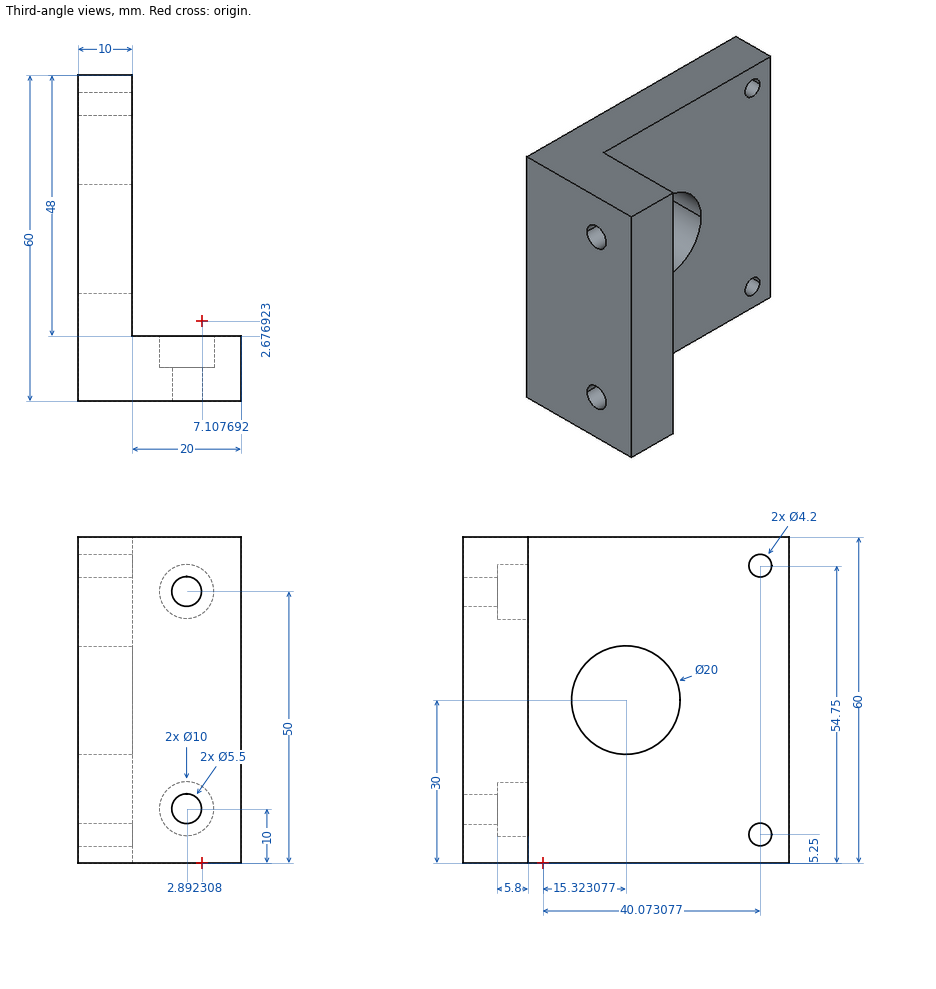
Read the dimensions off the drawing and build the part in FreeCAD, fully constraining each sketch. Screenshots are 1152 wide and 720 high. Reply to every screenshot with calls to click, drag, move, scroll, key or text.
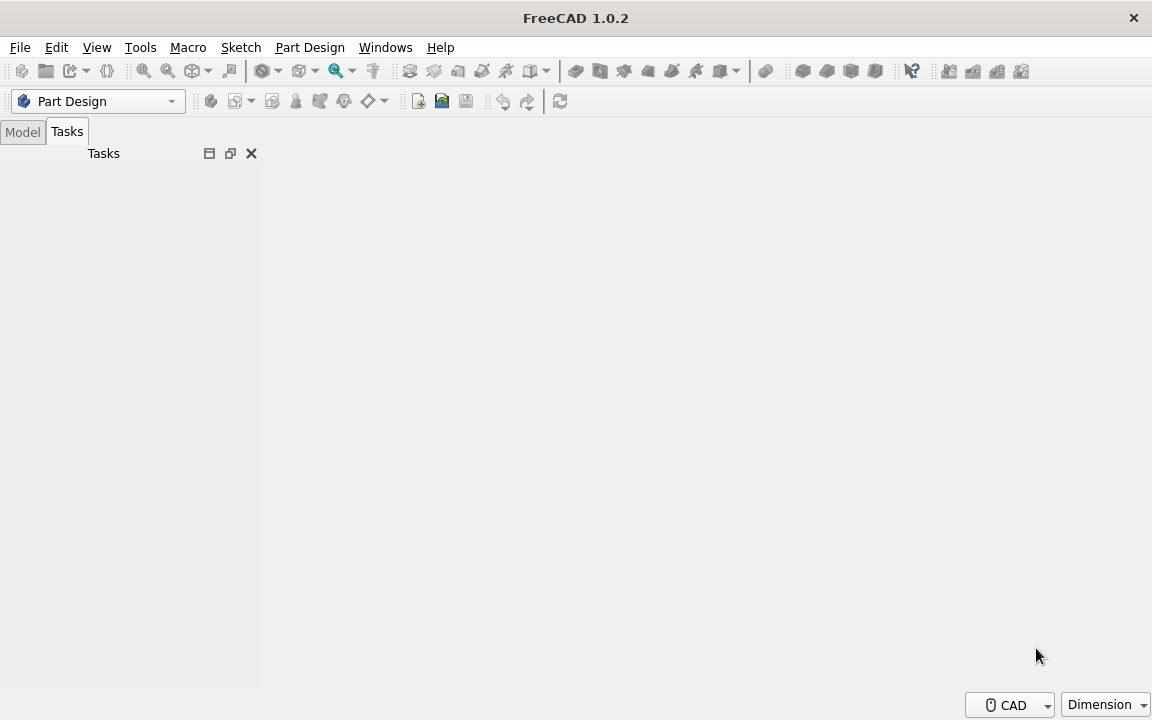
click(418, 102)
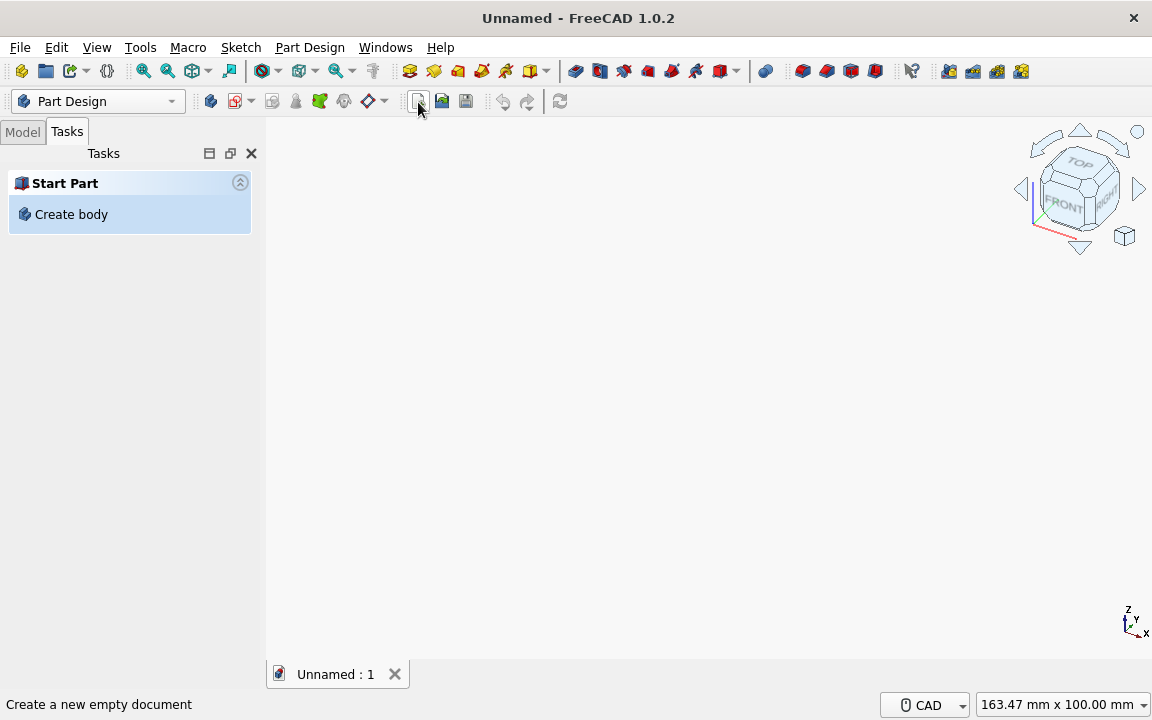
click(236, 102)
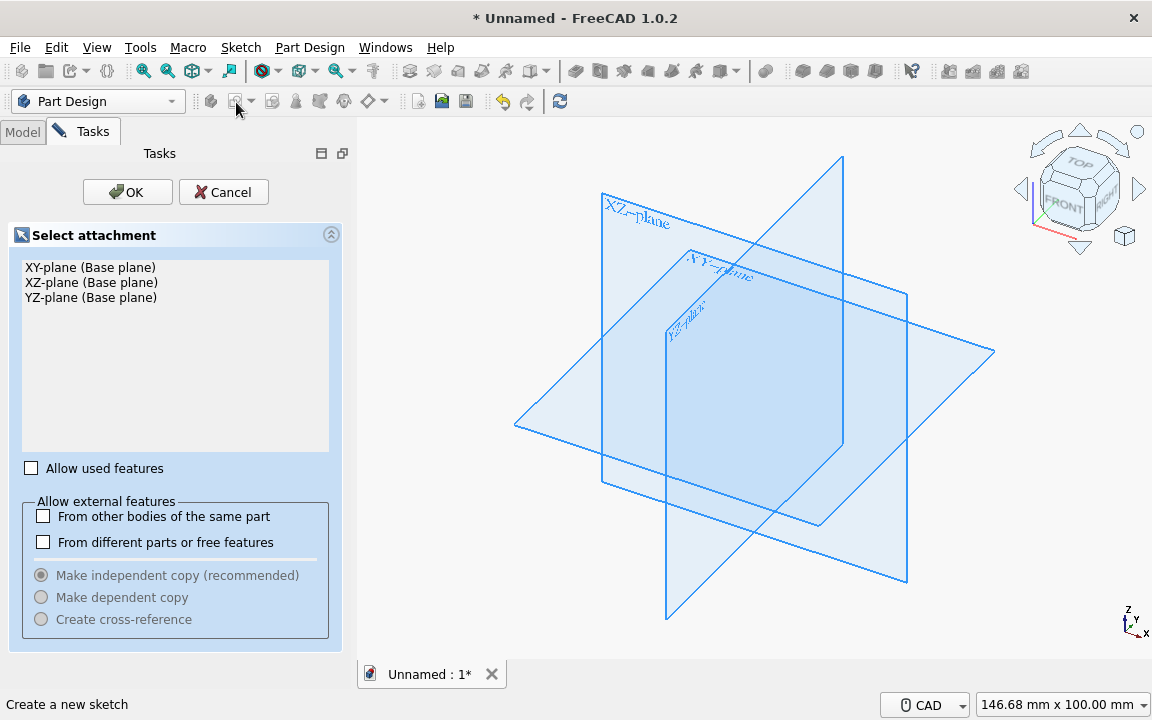
click(82, 268)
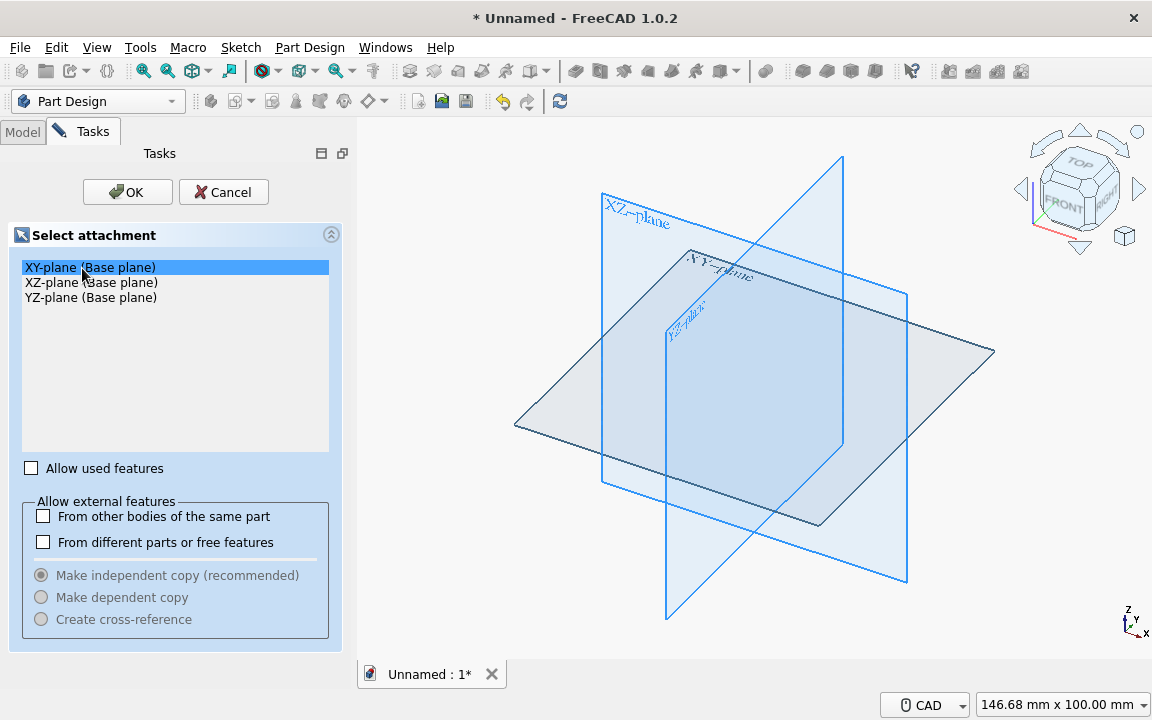
click(128, 192)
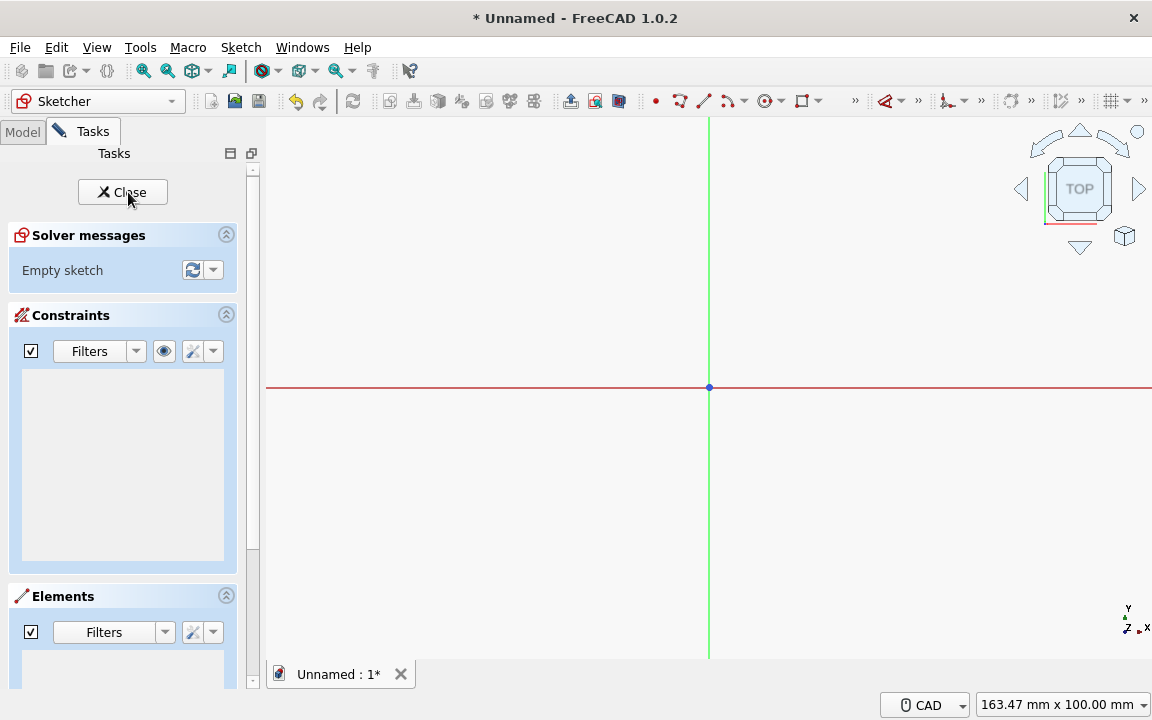
scroll(524, 631, down, 1)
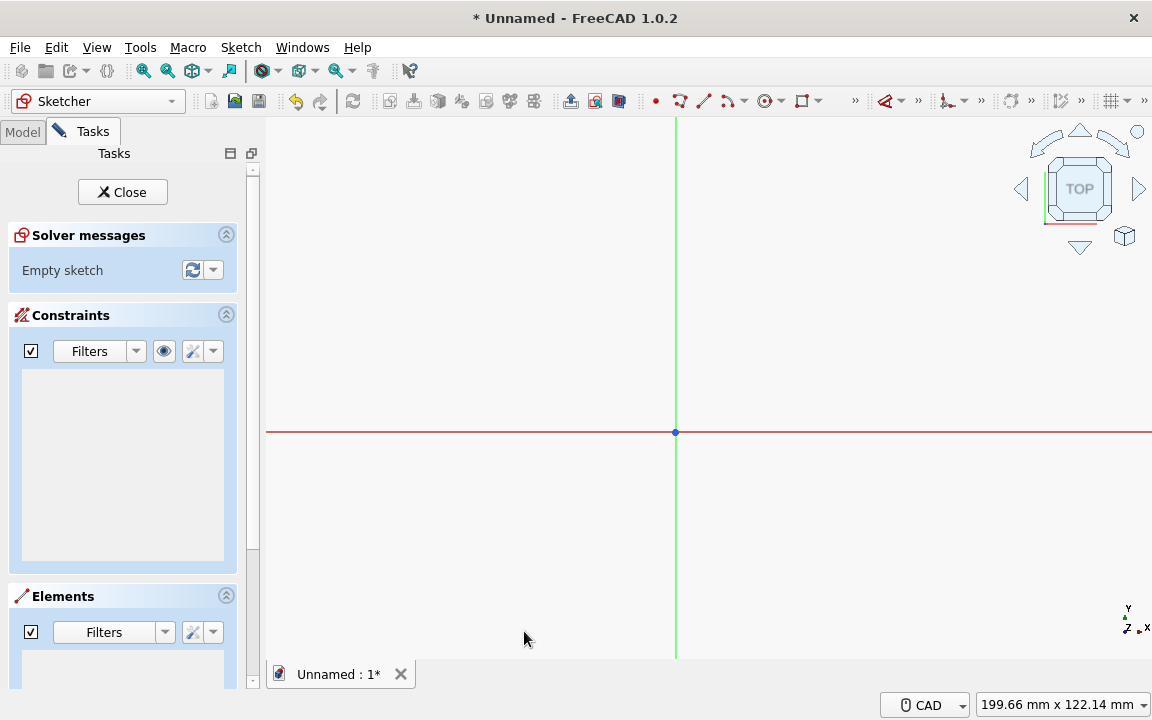
click(680, 102)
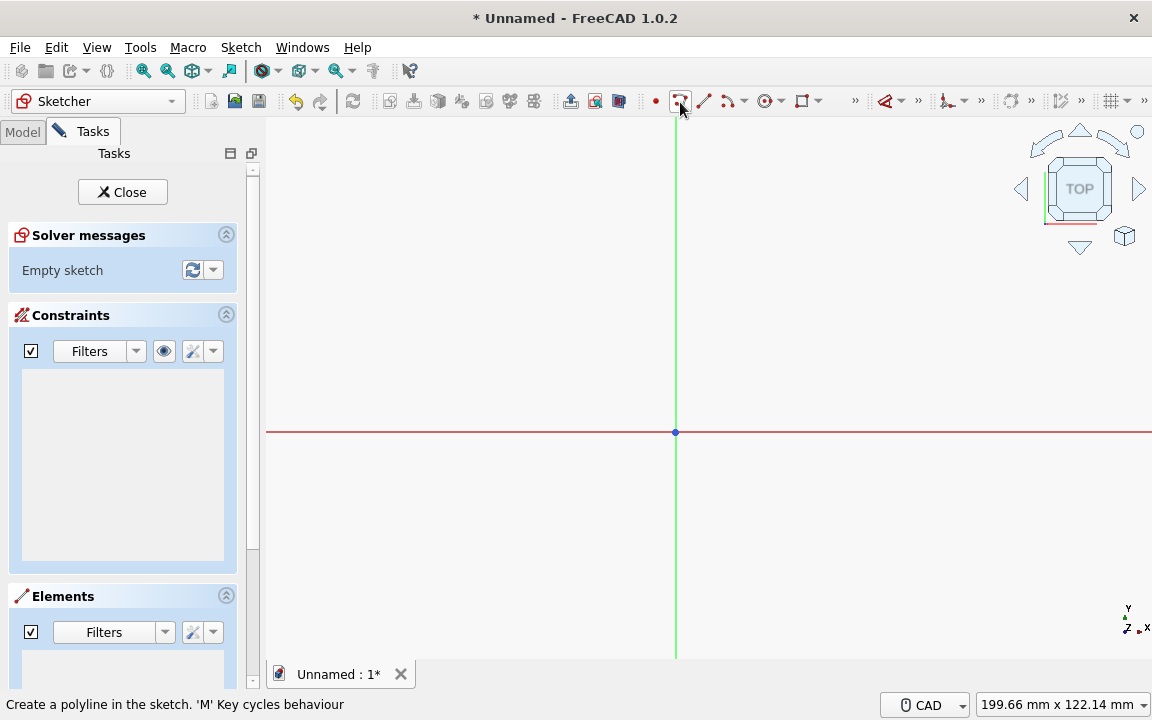
scroll(707, 444, up, 2)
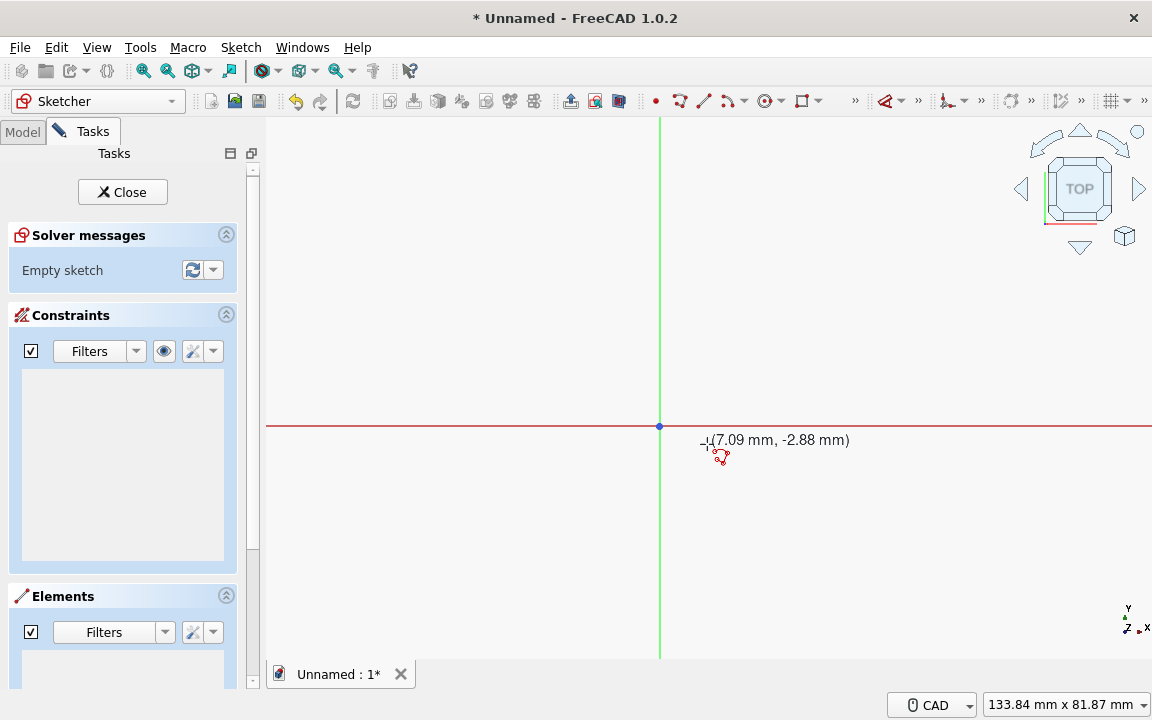
click(707, 444)
click(574, 444)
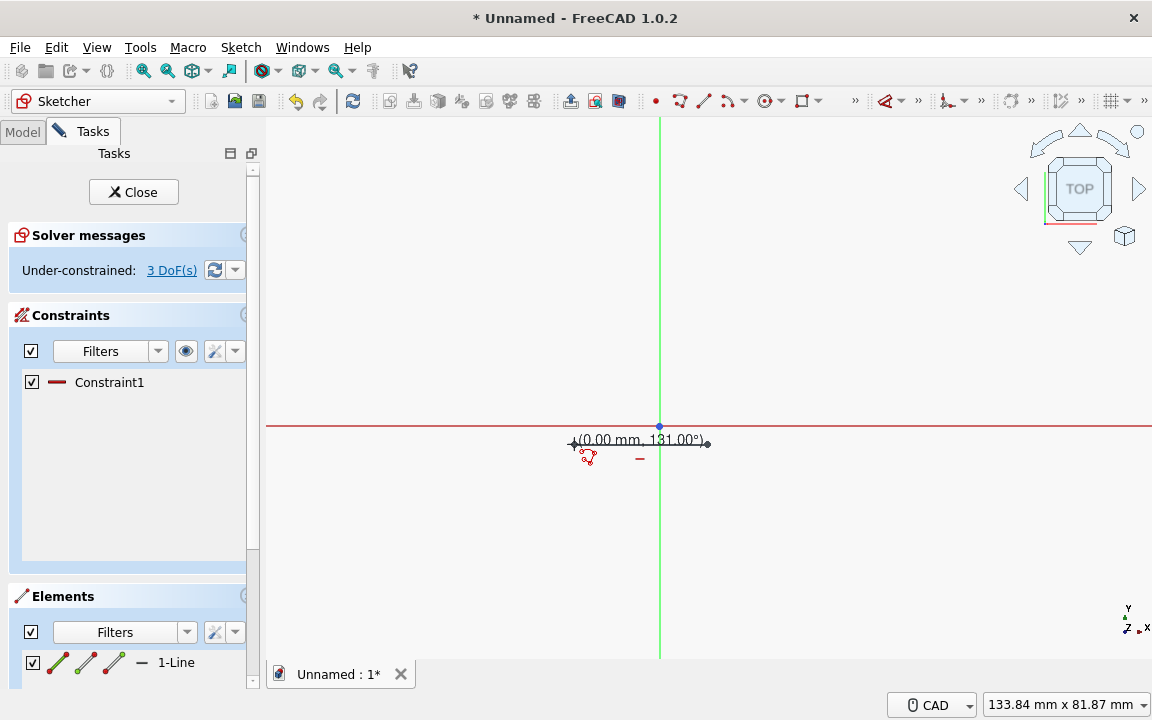
scroll(789, 631, down, 1)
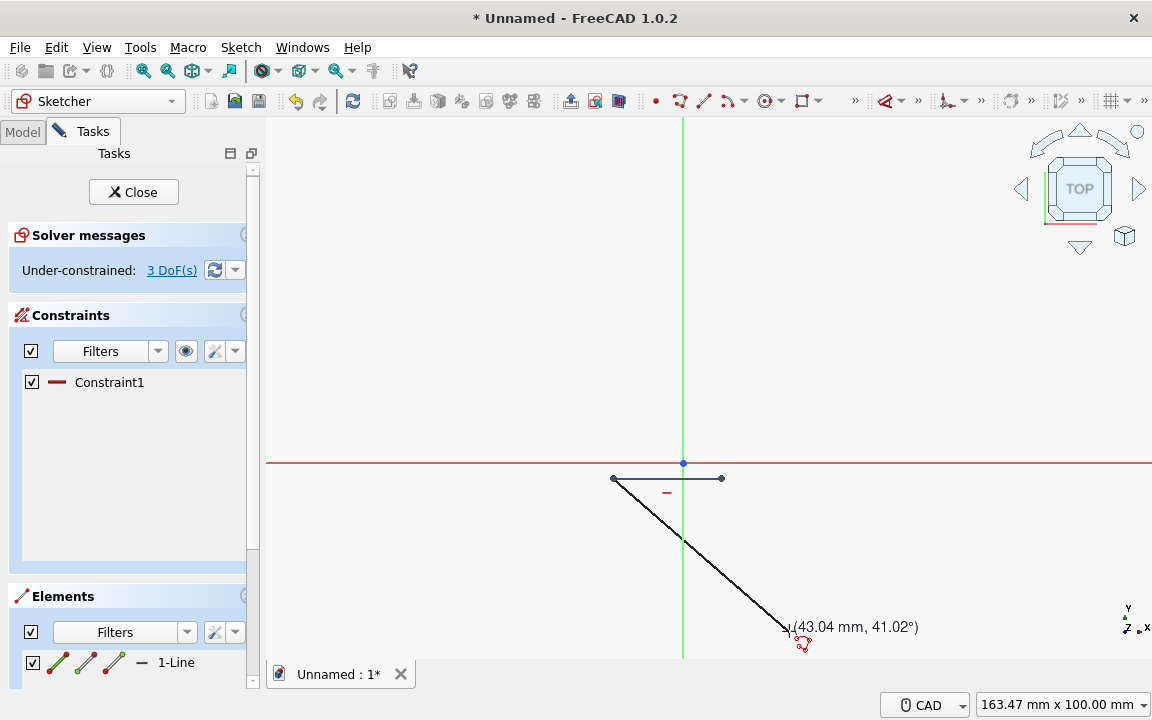
click(613, 218)
click(559, 218)
click(559, 543)
click(722, 543)
click(722, 479)
key(Escape)
key(Escape)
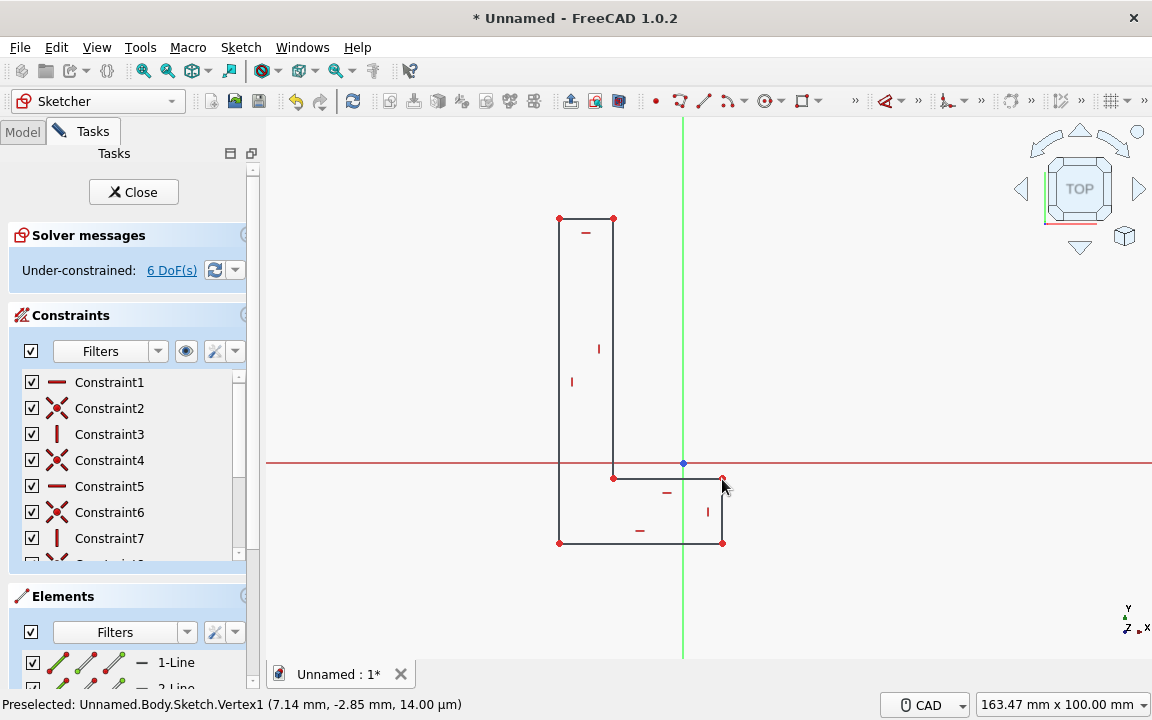
click(646, 479)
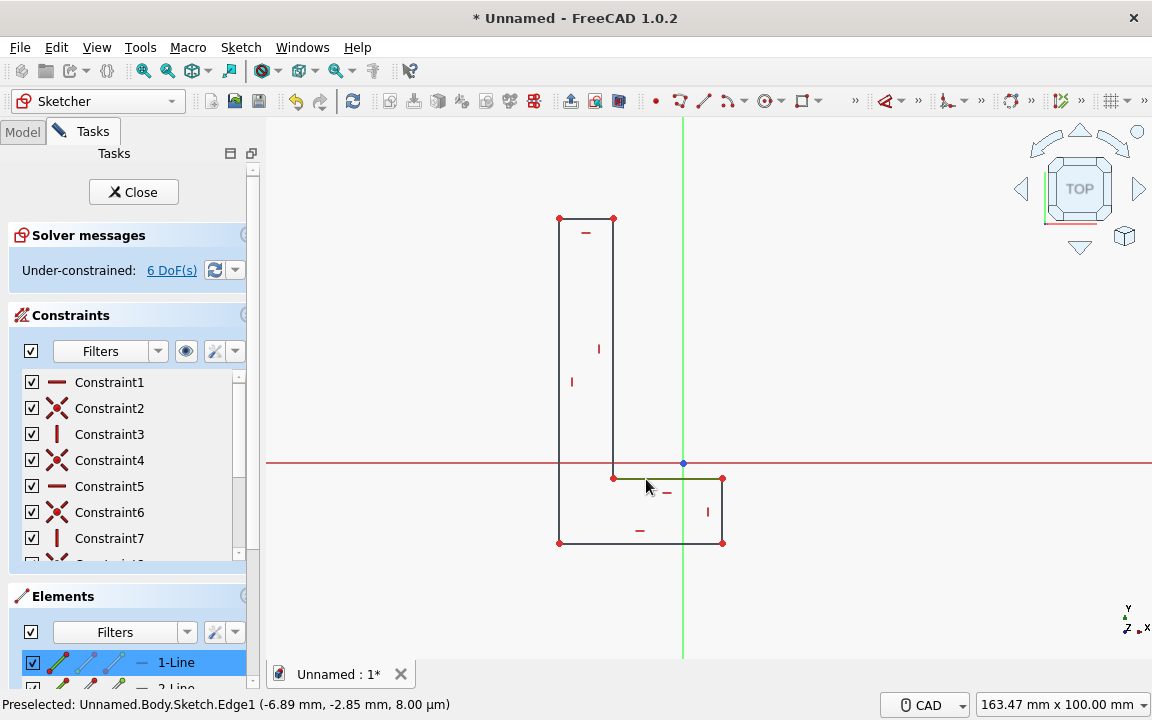
key(l)